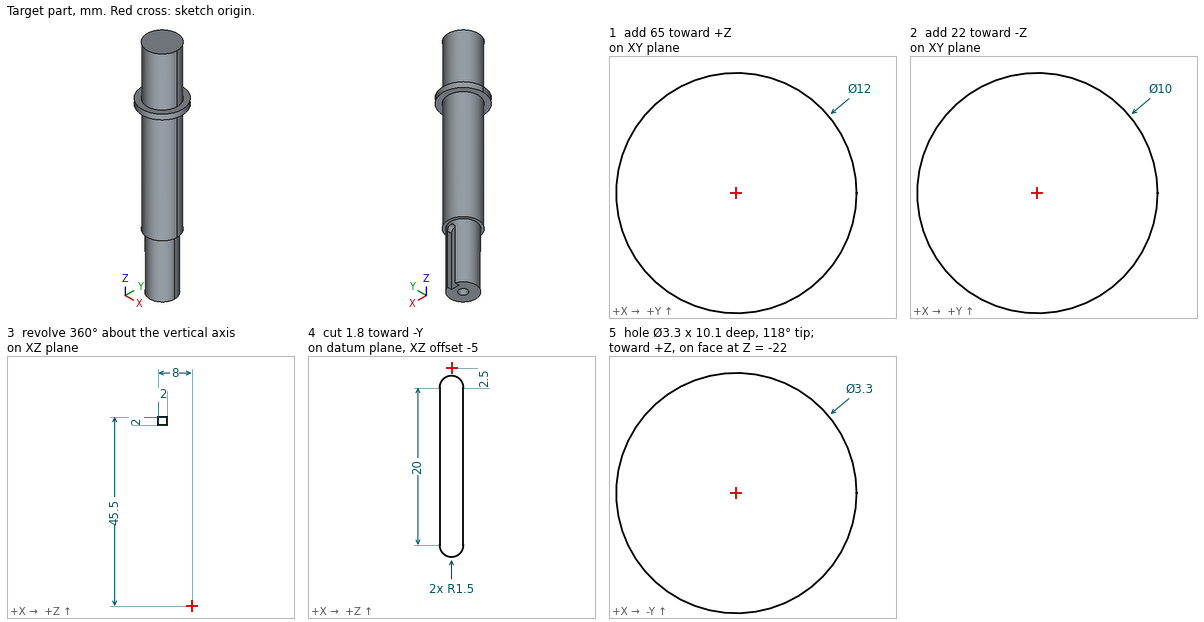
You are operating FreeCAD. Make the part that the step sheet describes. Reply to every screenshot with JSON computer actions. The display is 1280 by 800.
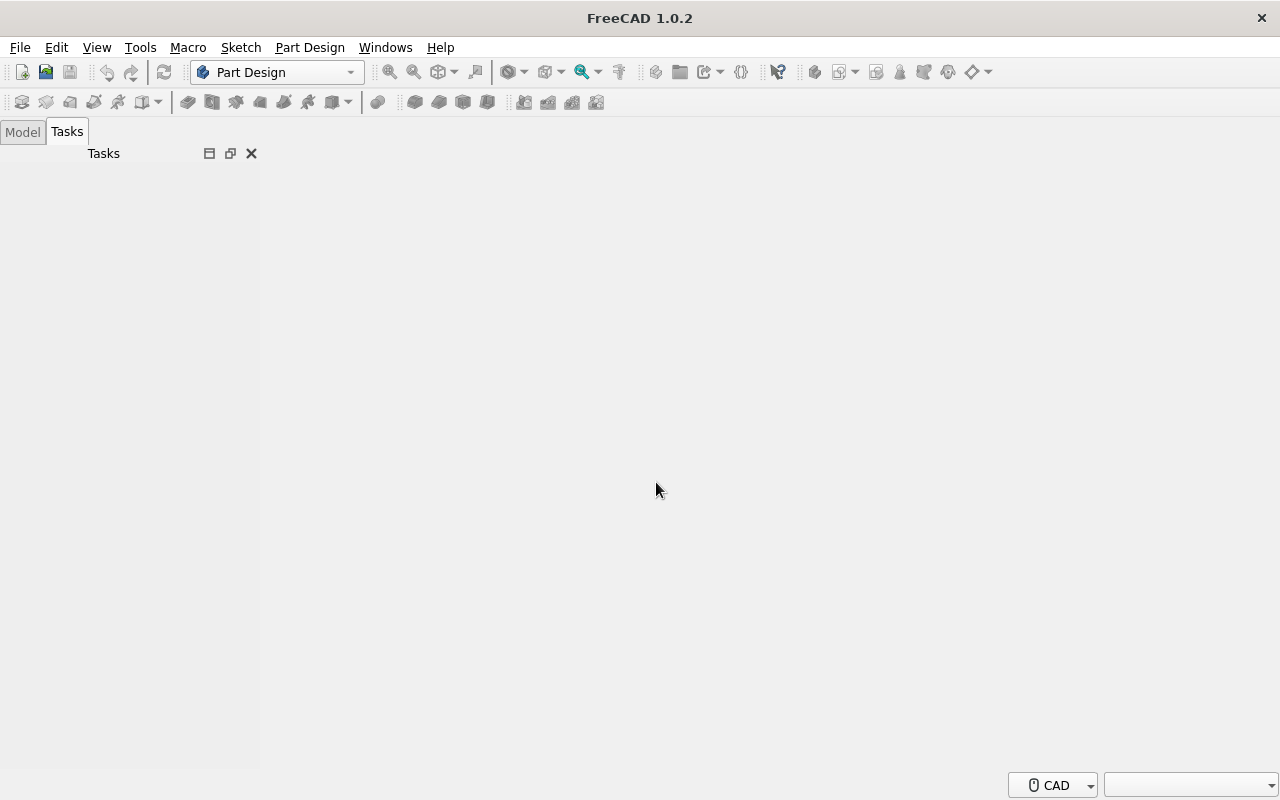
{"action": "left_click", "coordinate": [22, 72]}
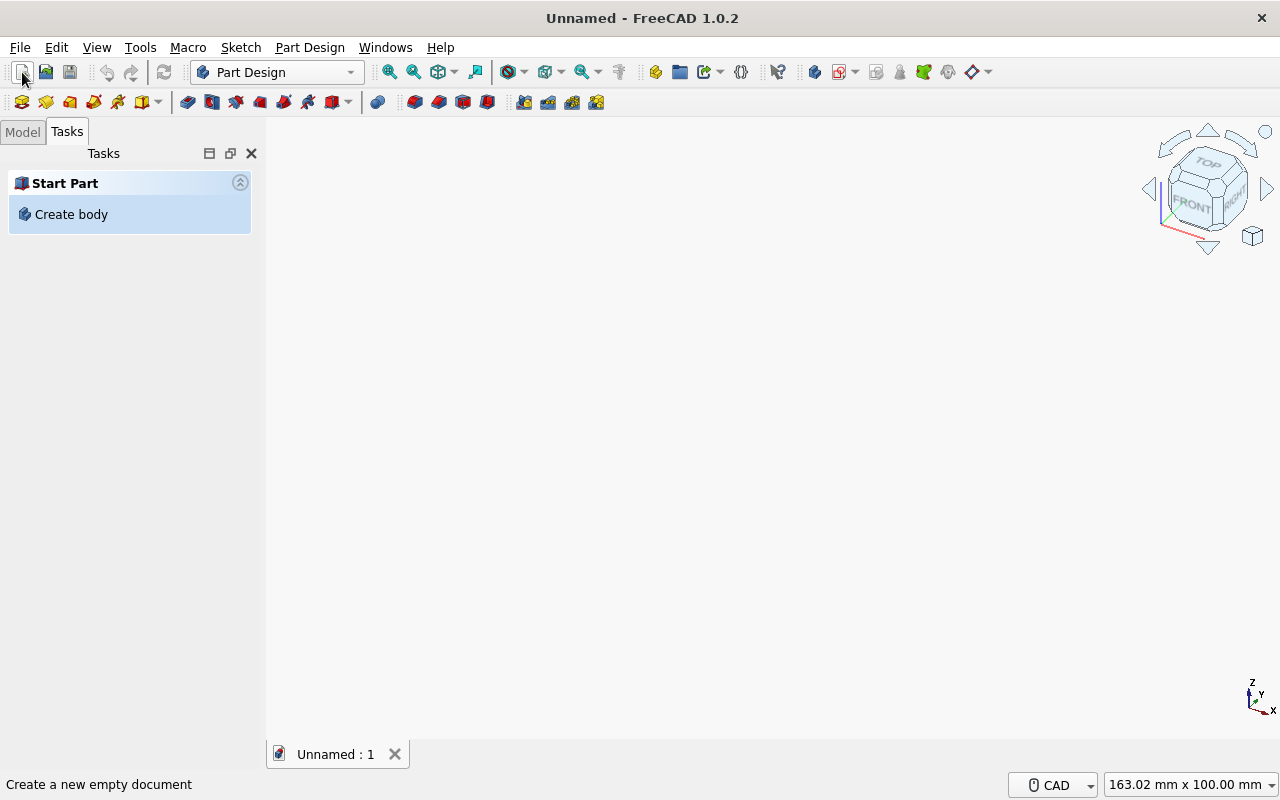
{"action": "left_click", "coordinate": [840, 72]}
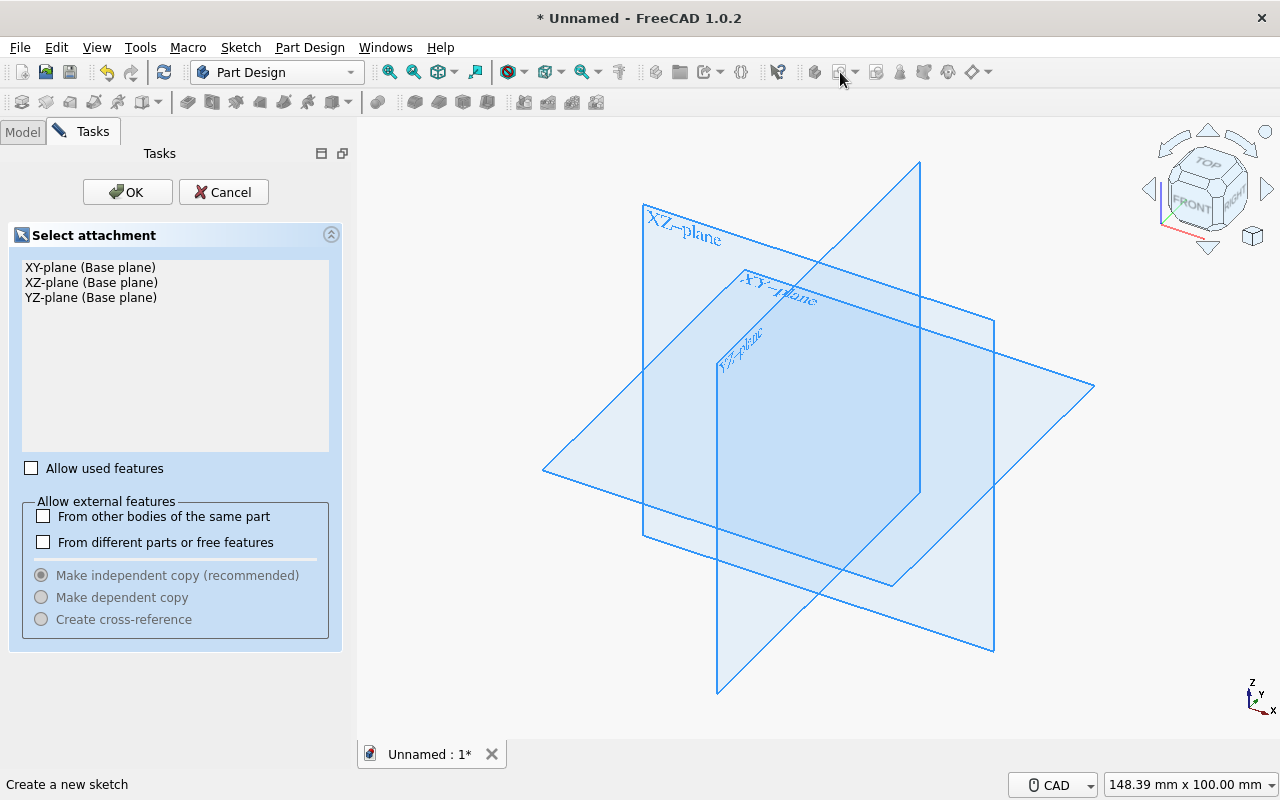
{"action": "left_click", "coordinate": [82, 268]}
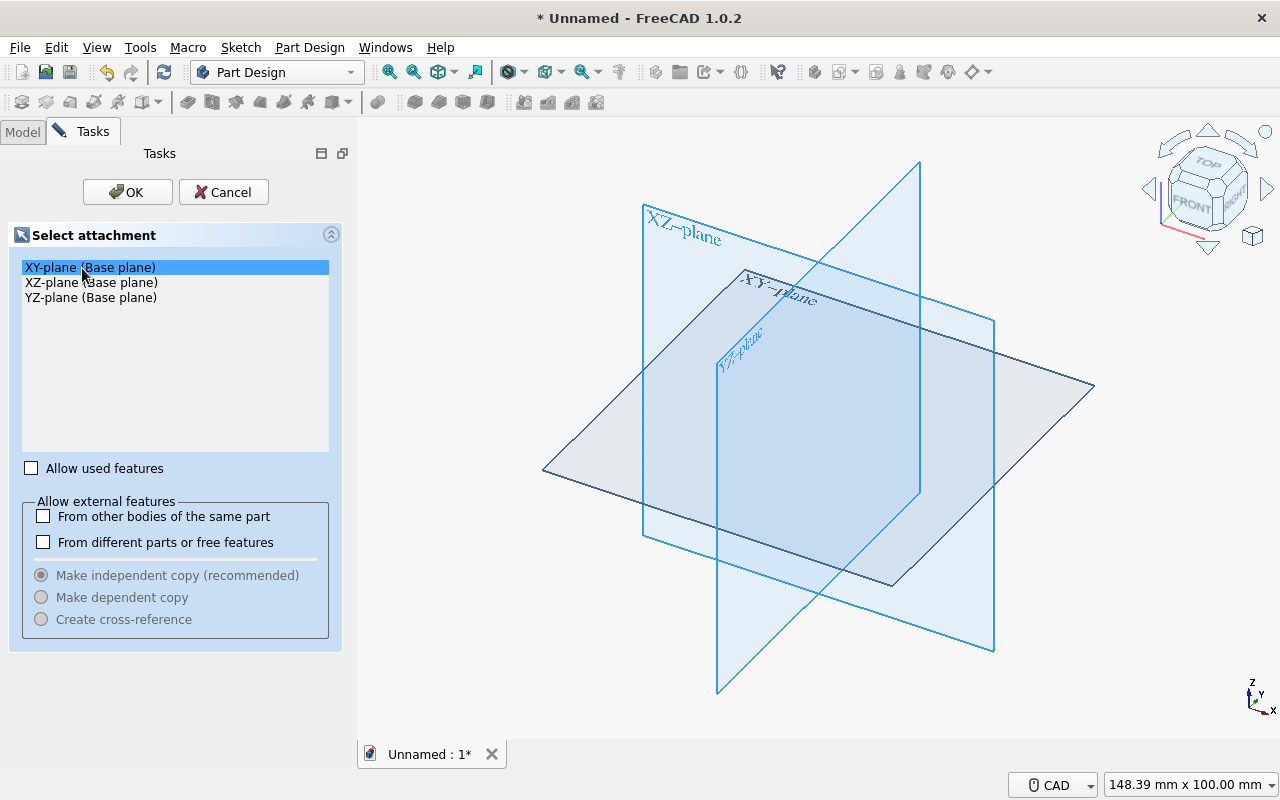
{"action": "left_click", "coordinate": [128, 192]}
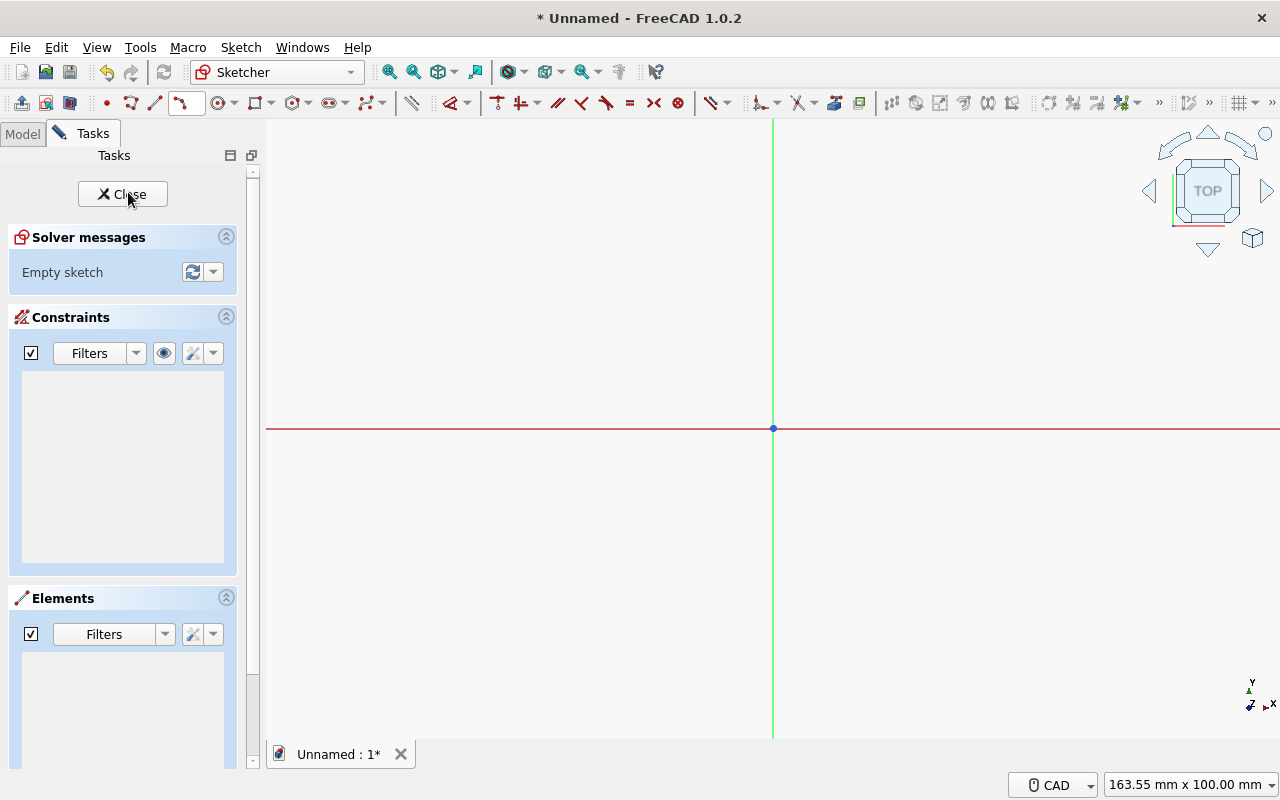
{"action": "scroll", "coordinate": [790, 429], "scroll_direction": "up", "scroll_amount": 8}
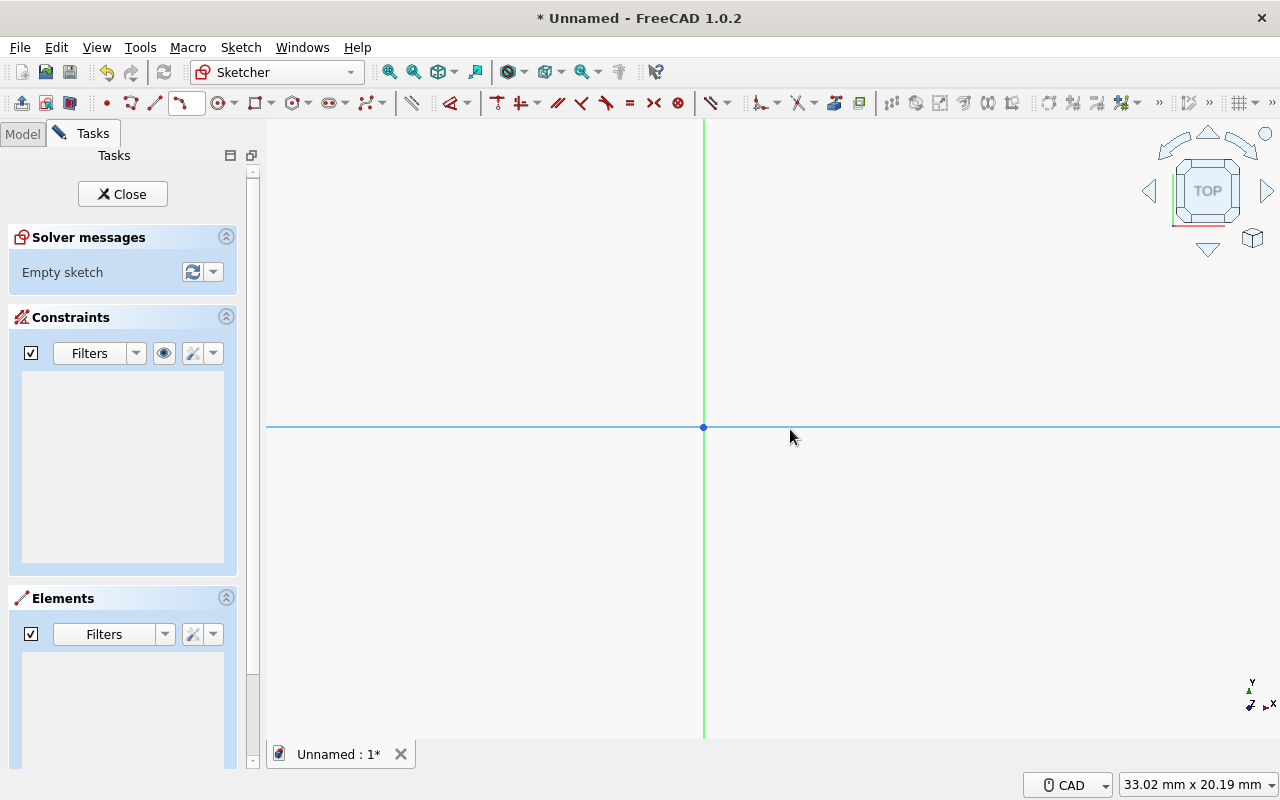
{"action": "left_click", "coordinate": [218, 104]}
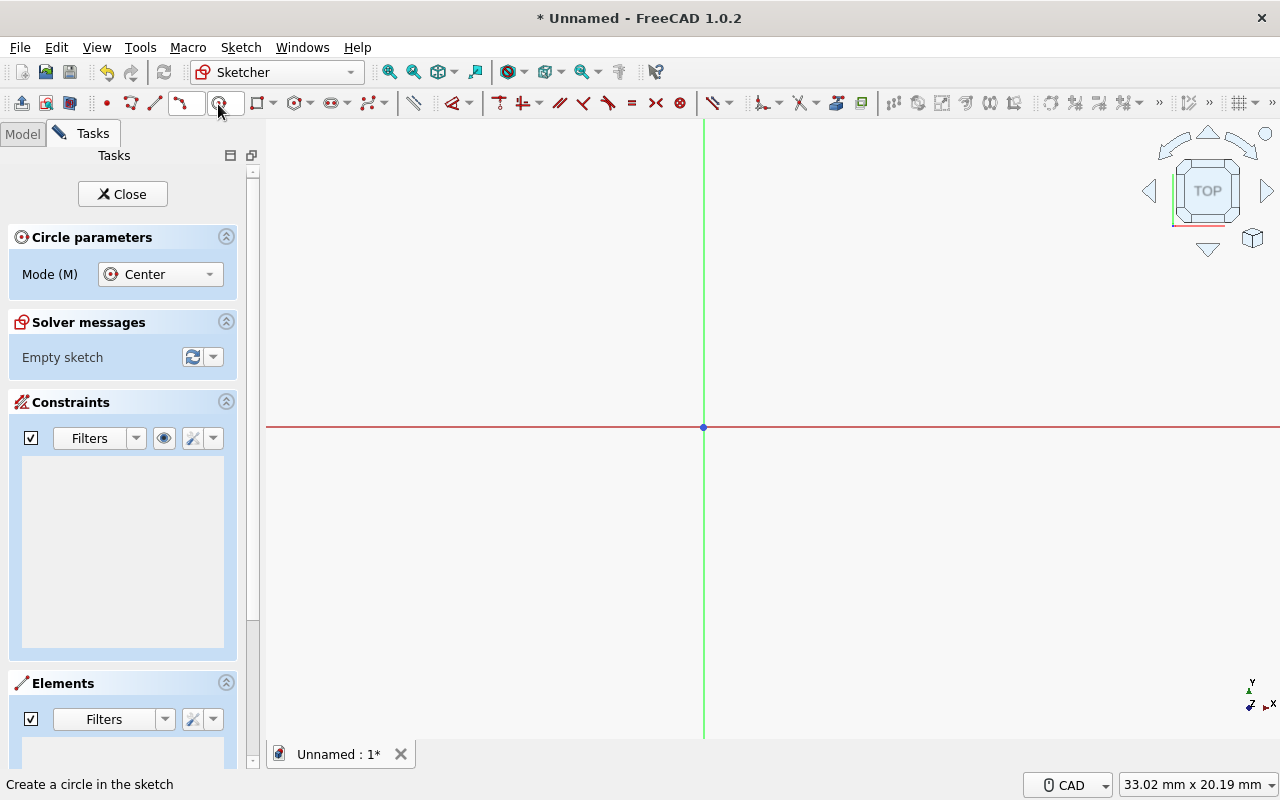
{"action": "left_click", "coordinate": [704, 427]}
{"action": "mouse_move", "coordinate": [834, 297]}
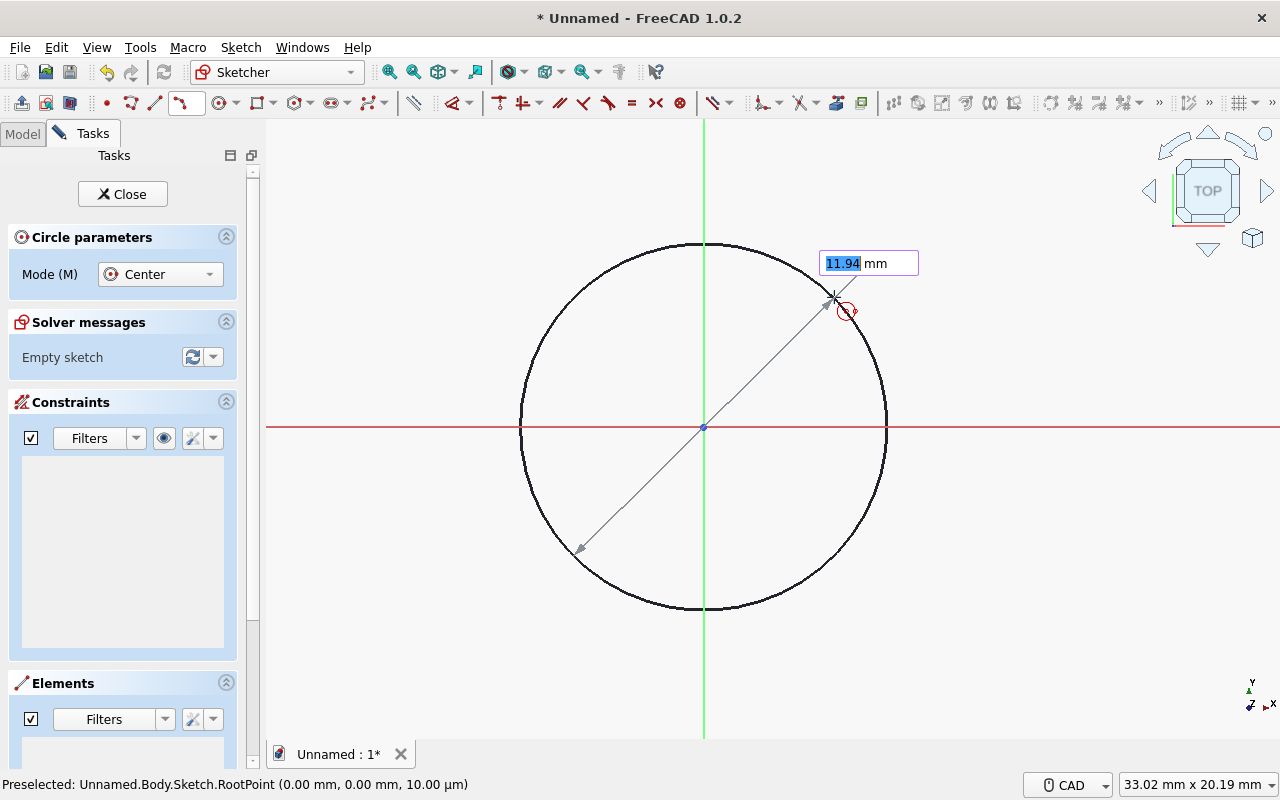
{"action": "type", "text": "12"}
{"action": "key", "text": "Return"}
{"action": "key", "text": "Escape"}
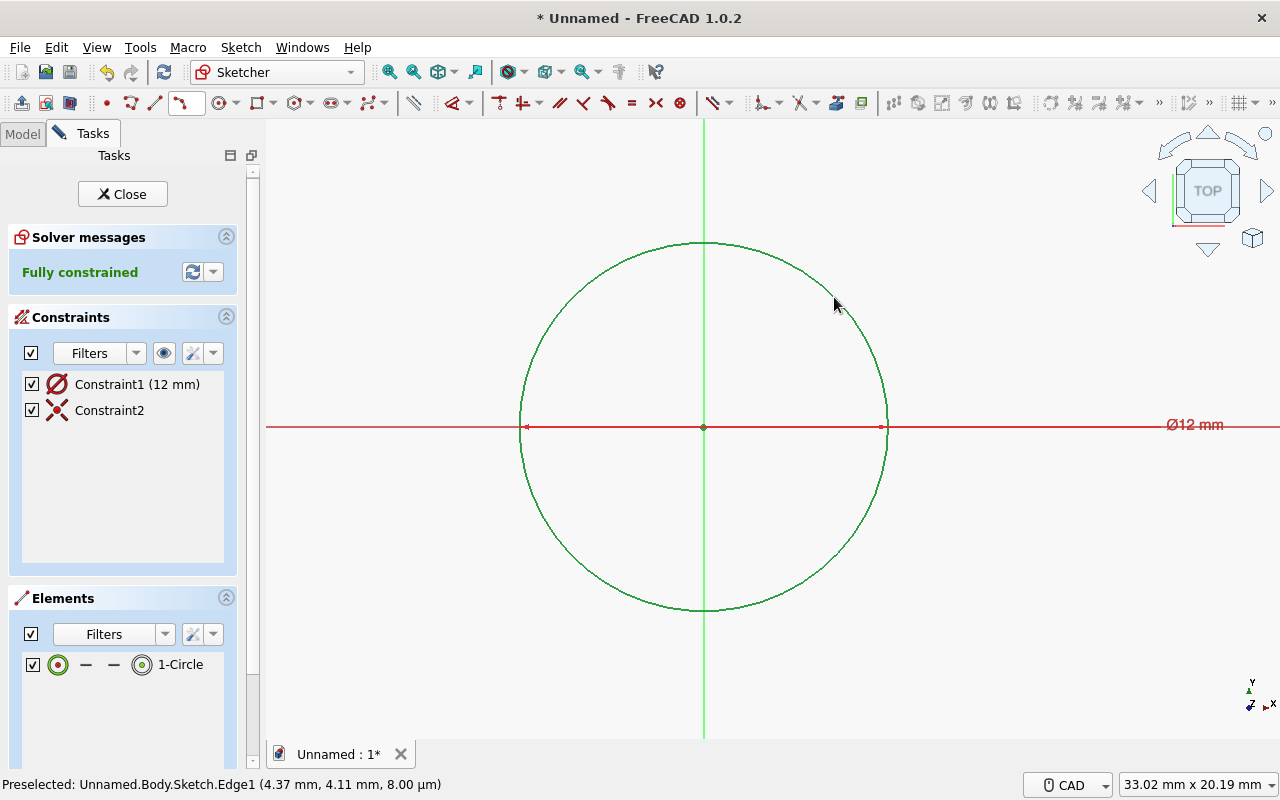
{"action": "left_click", "coordinate": [123, 194]}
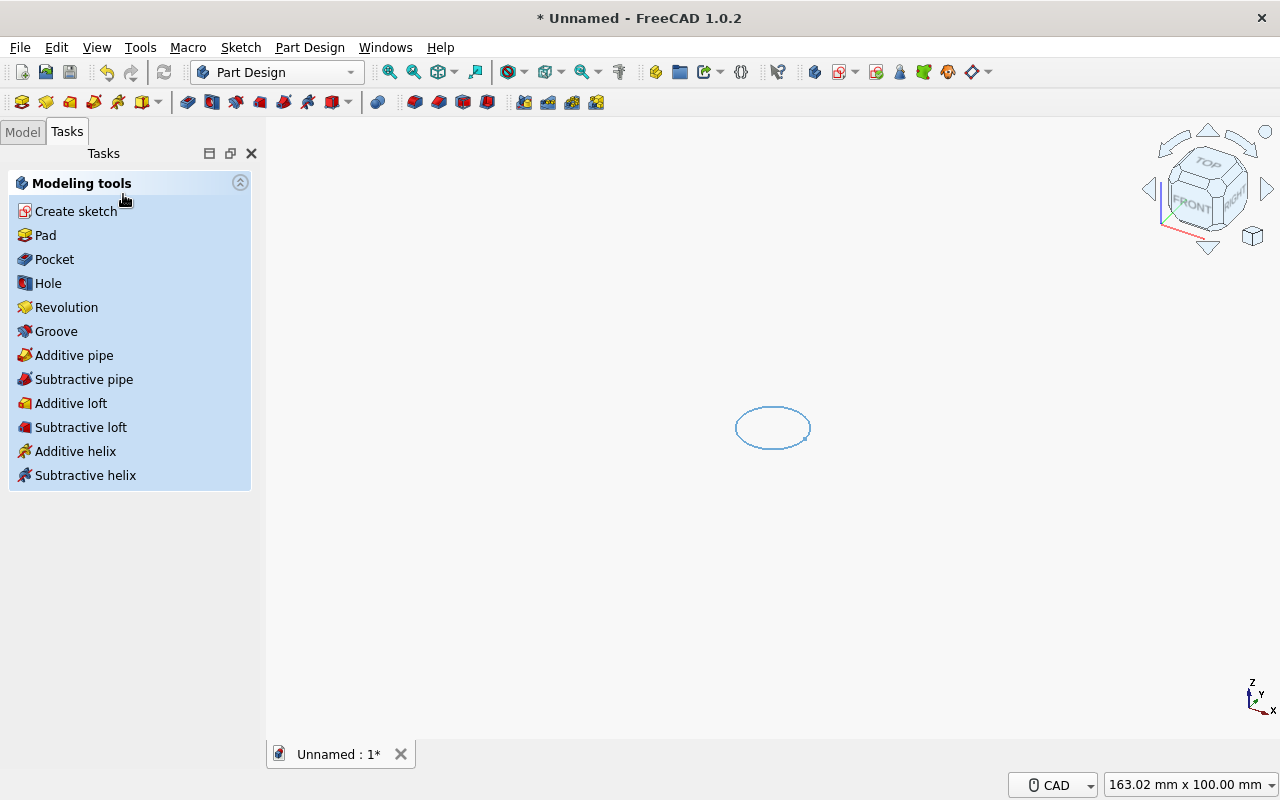
{"action": "left_click", "coordinate": [22, 102]}